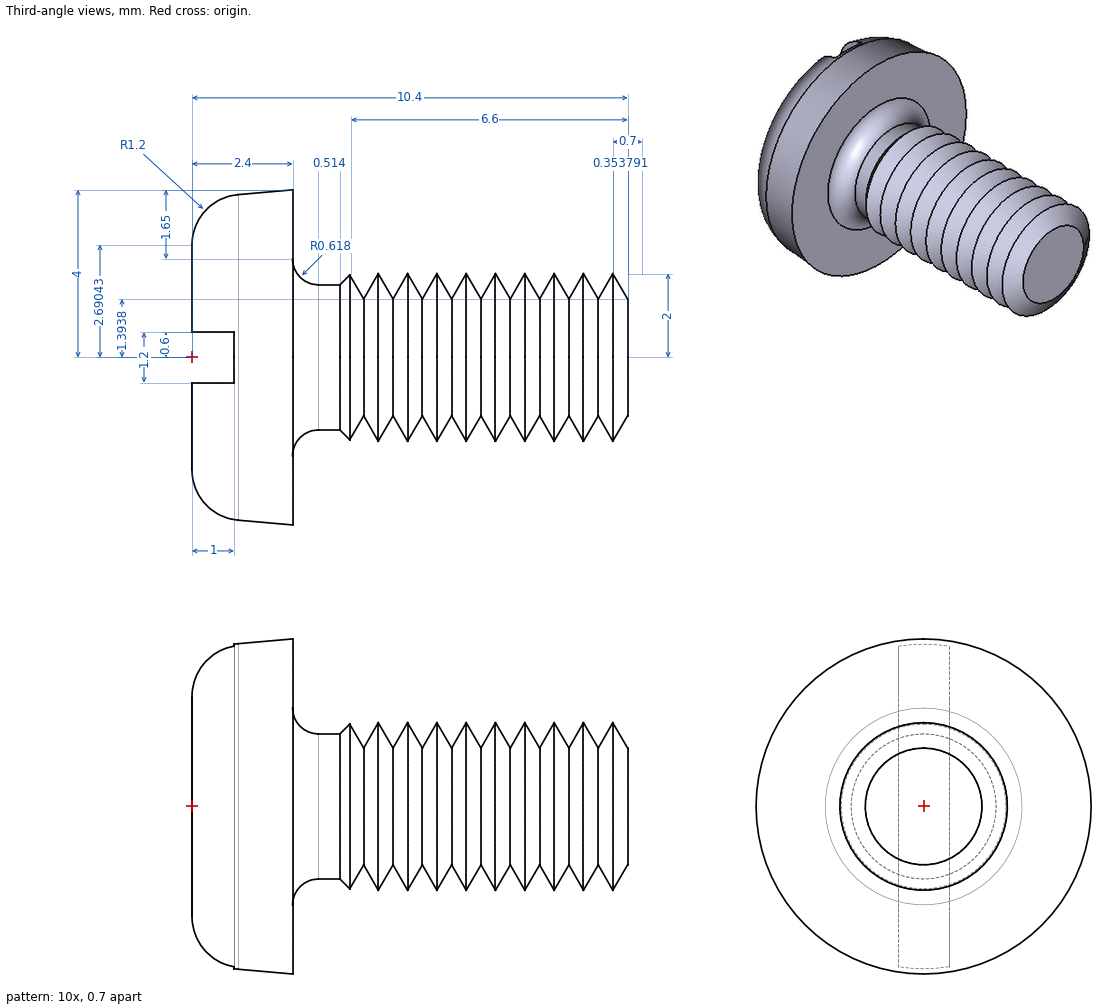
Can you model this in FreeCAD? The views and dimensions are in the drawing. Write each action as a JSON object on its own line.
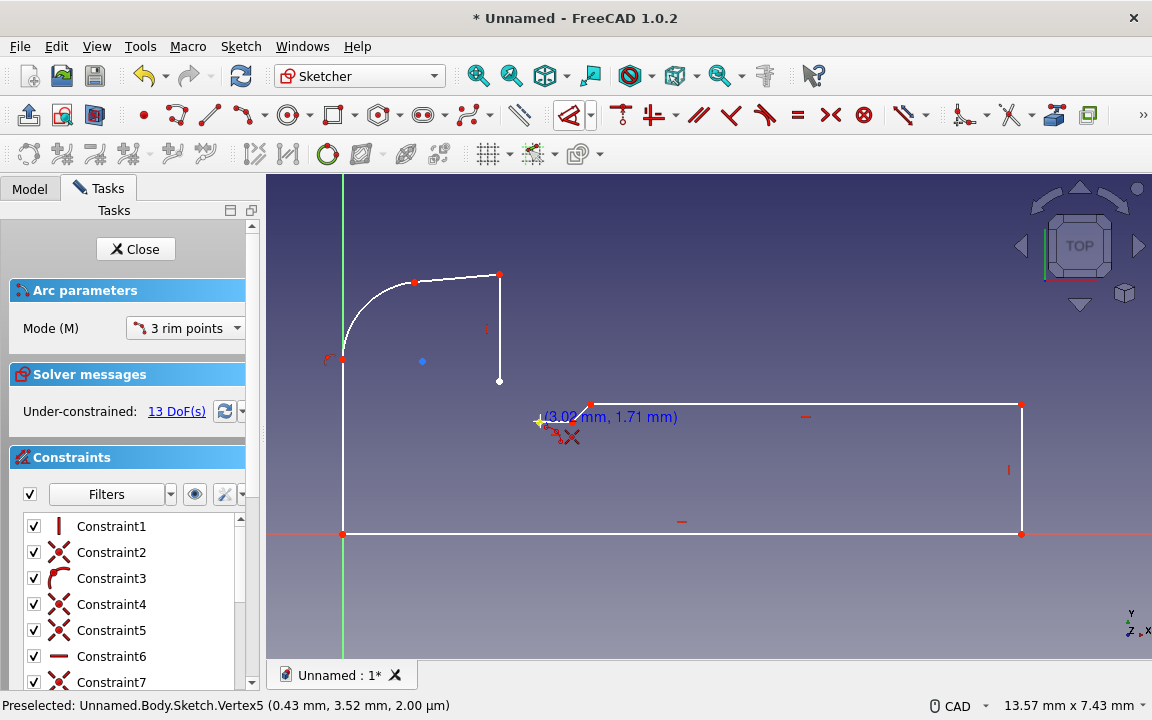
{"action": "left_click", "coordinate": [540, 422]}
{"action": "left_click", "coordinate": [500, 382]}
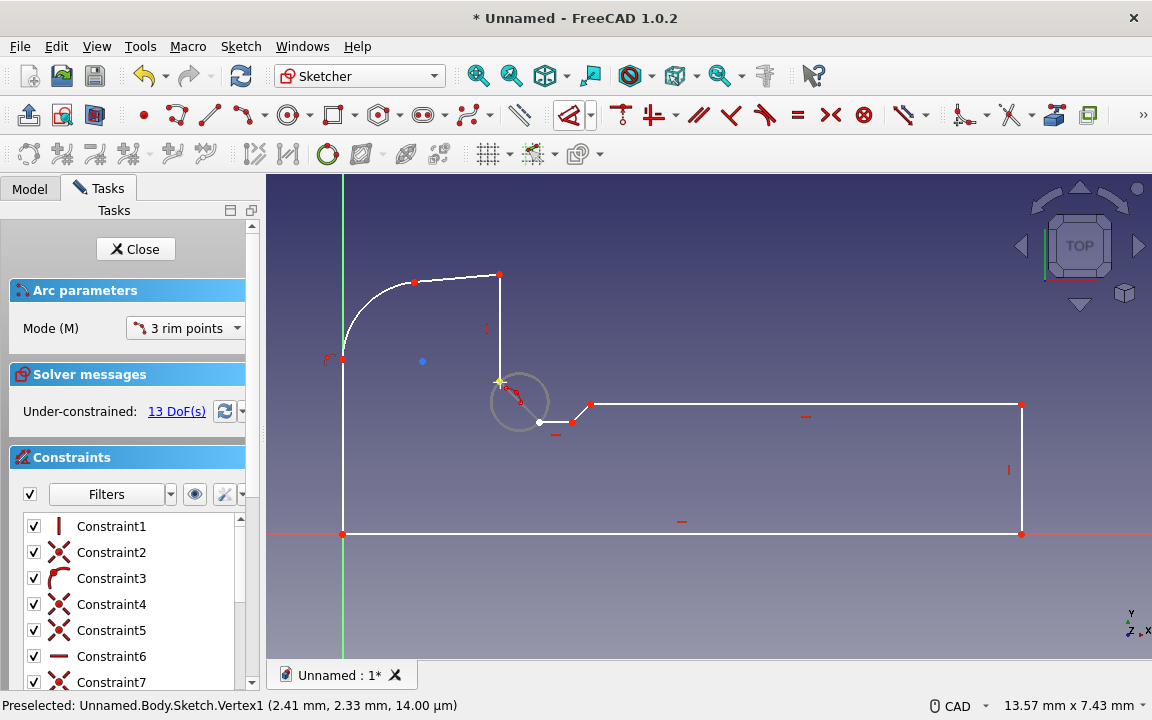
{"action": "scroll", "coordinate": [511, 409], "scroll_direction": "up", "scroll_amount": 2}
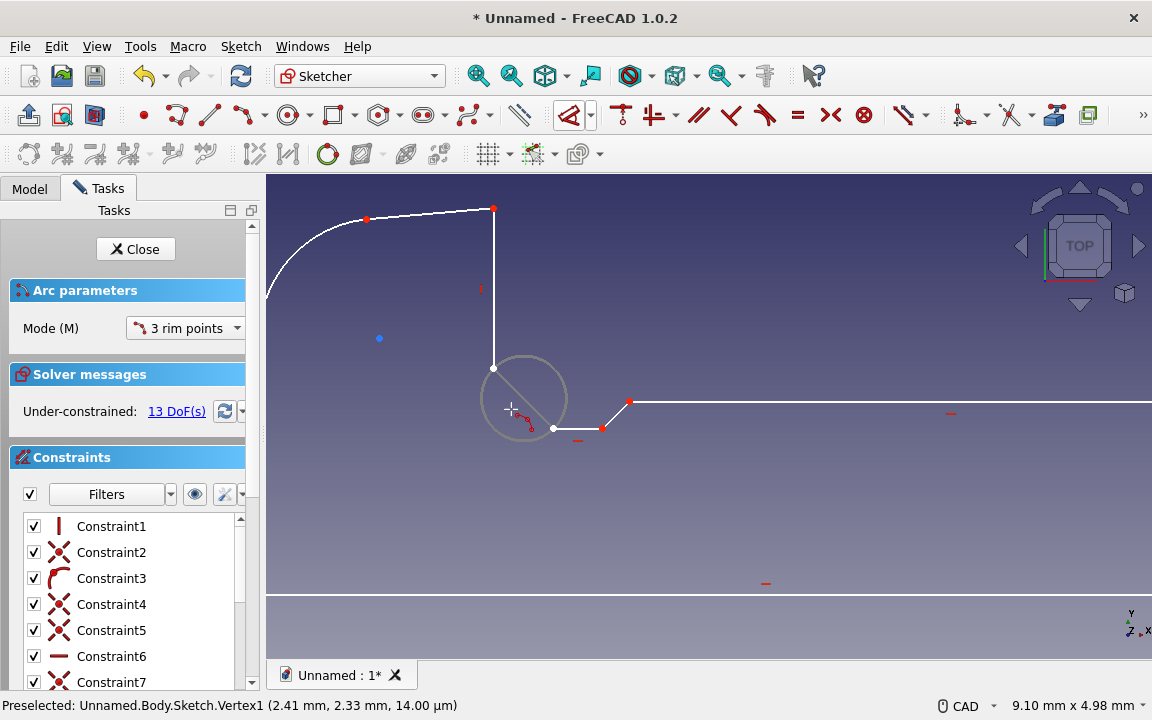
{"action": "left_click", "coordinate": [511, 409]}
{"action": "key", "text": "Escape"}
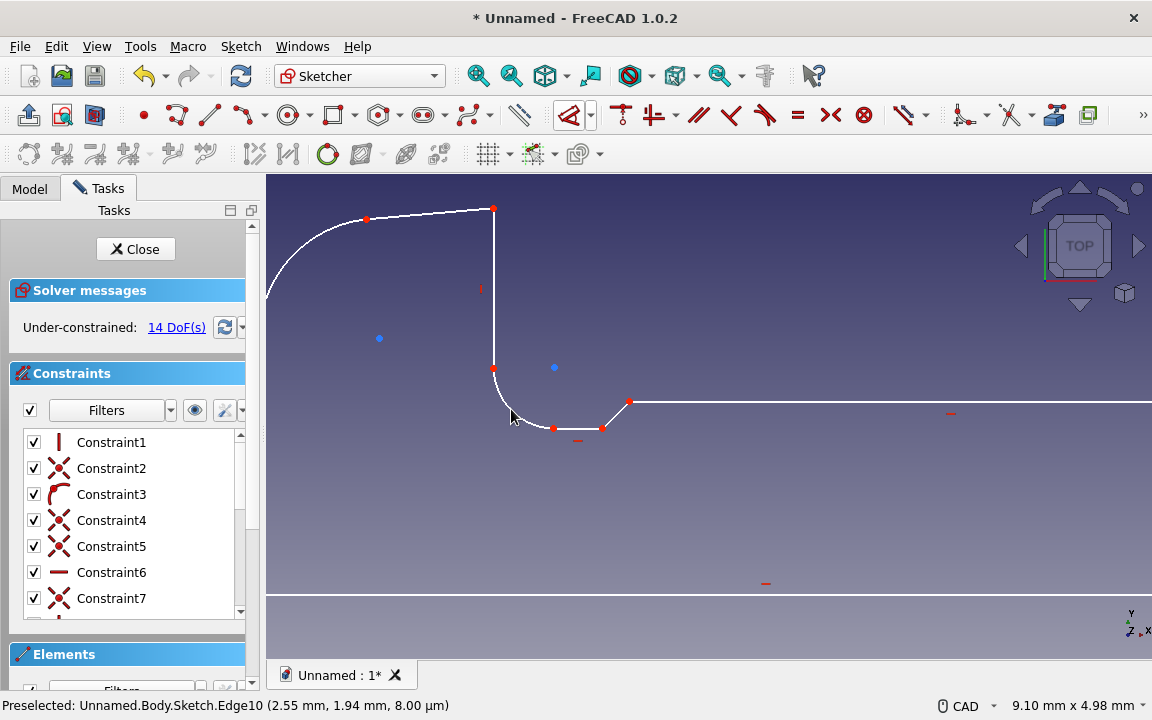
{"action": "left_click", "coordinate": [494, 320]}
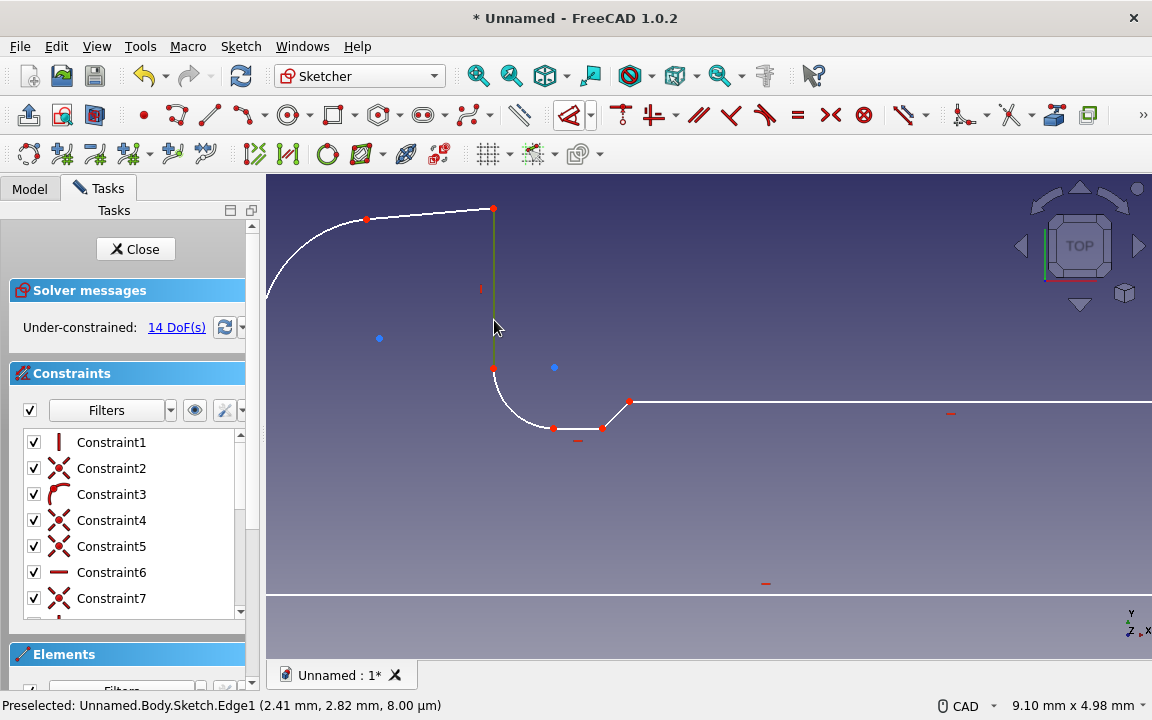
{"action": "left_click", "coordinate": [501, 396]}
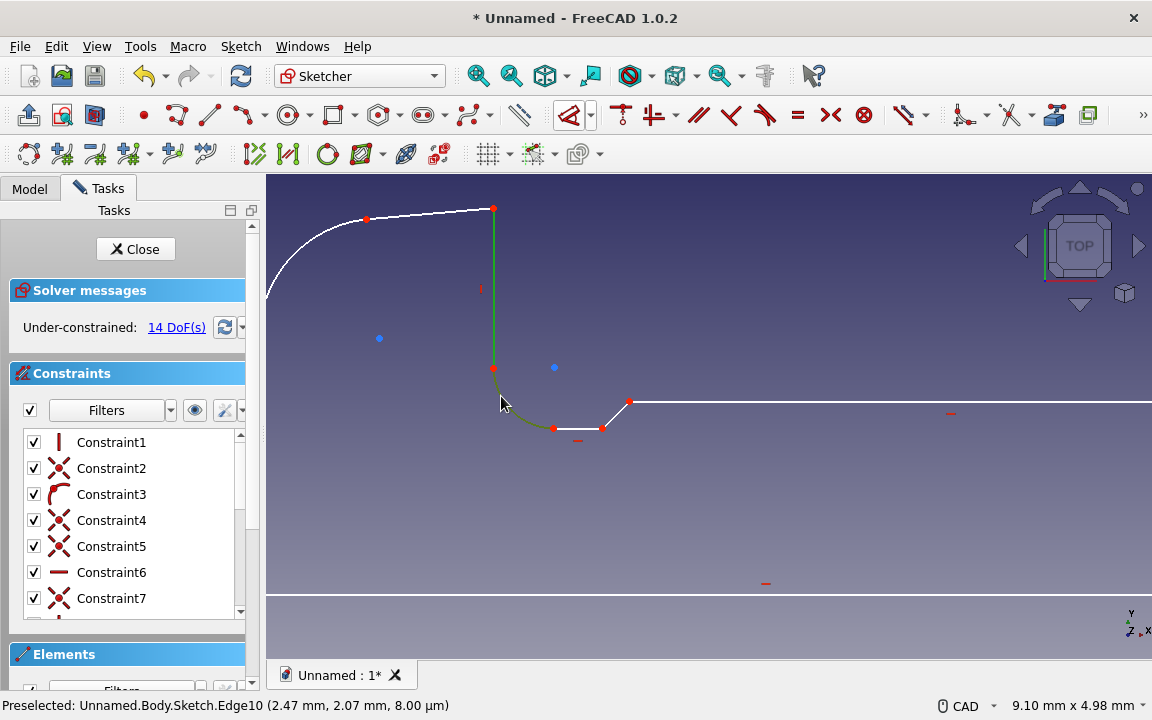
{"action": "left_click", "coordinate": [765, 116]}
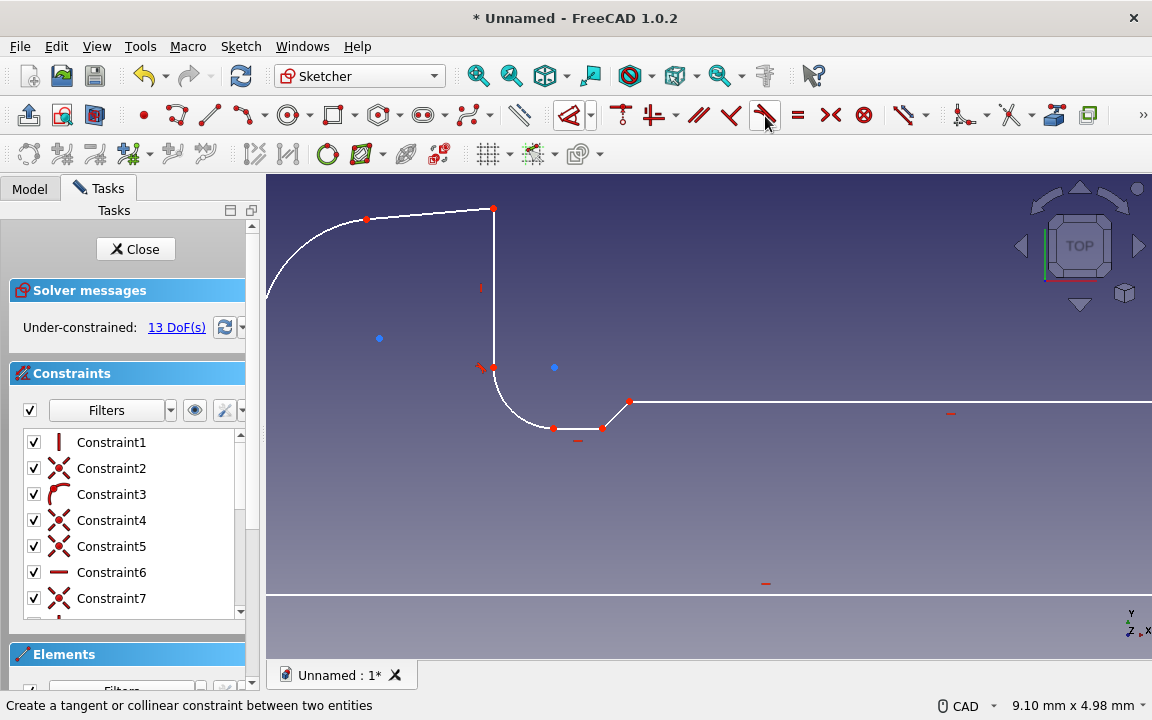
{"action": "left_click", "coordinate": [456, 212]}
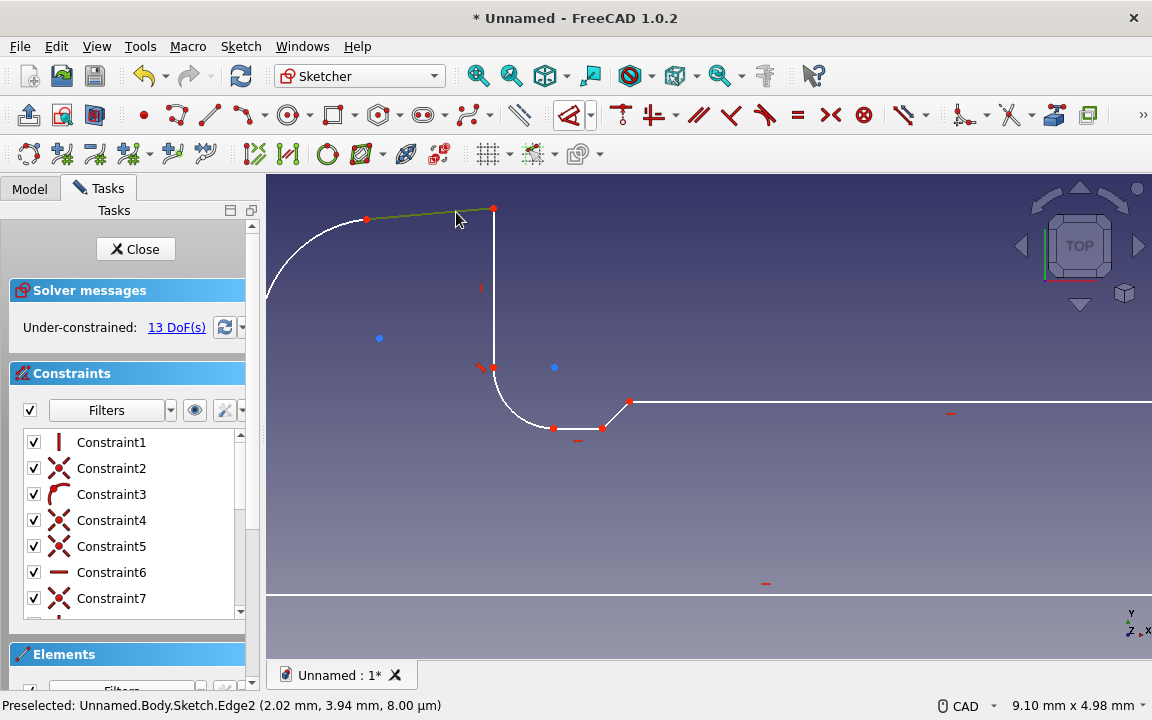
{"action": "left_click", "coordinate": [318, 235]}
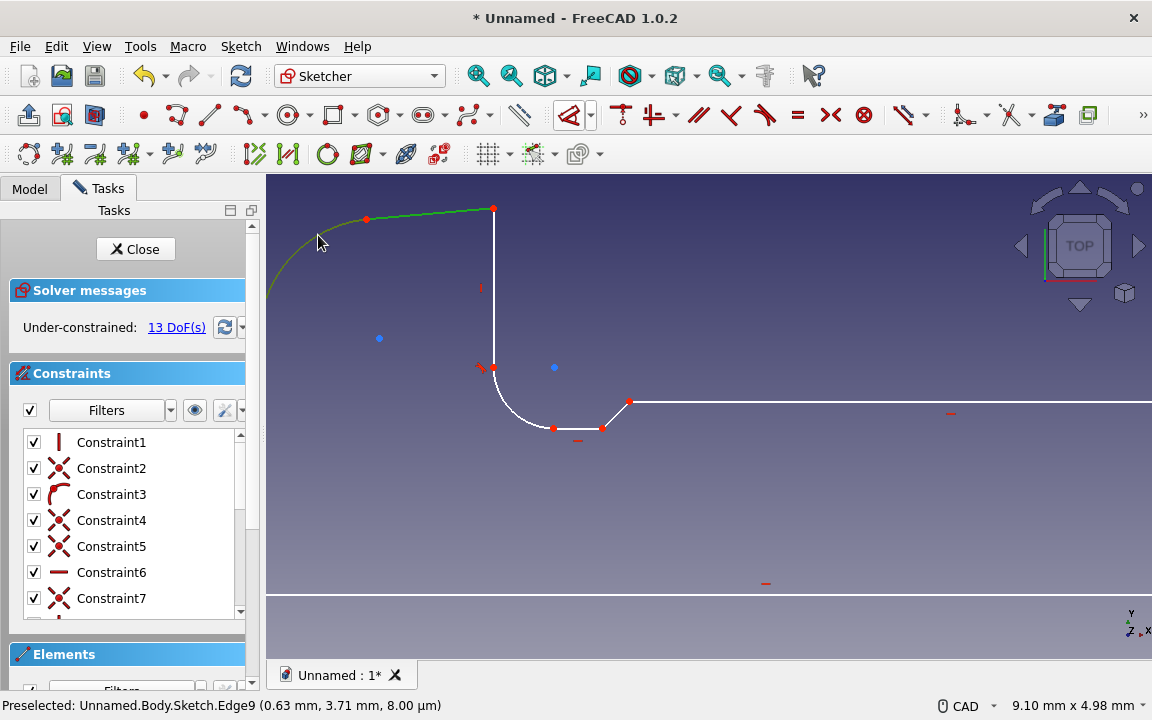
{"action": "left_click", "coordinate": [765, 116]}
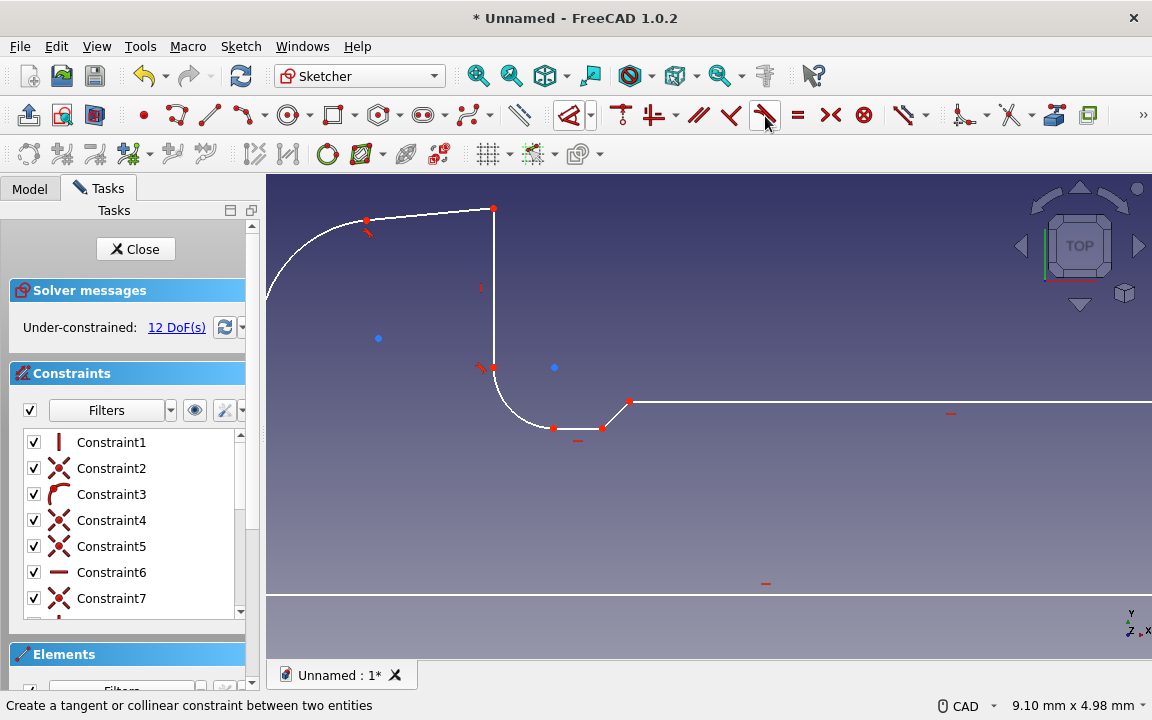
{"action": "scroll", "coordinate": [538, 430], "scroll_direction": "down", "scroll_amount": 4}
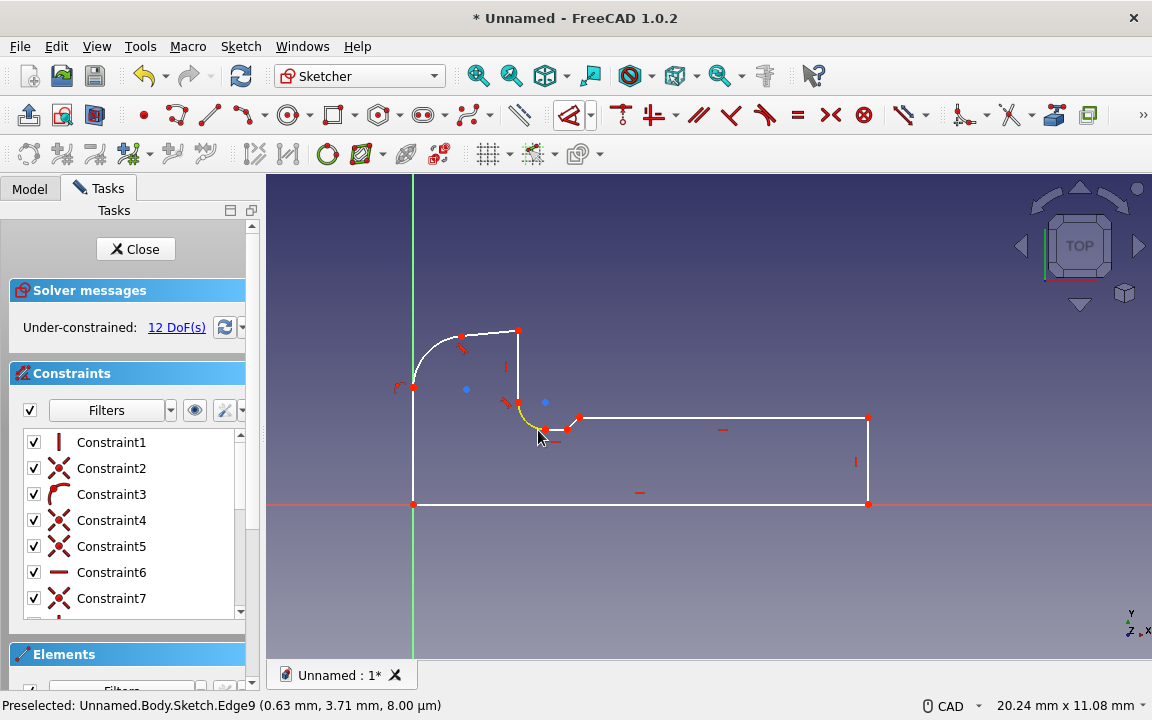
{"action": "left_click", "coordinate": [413, 423]}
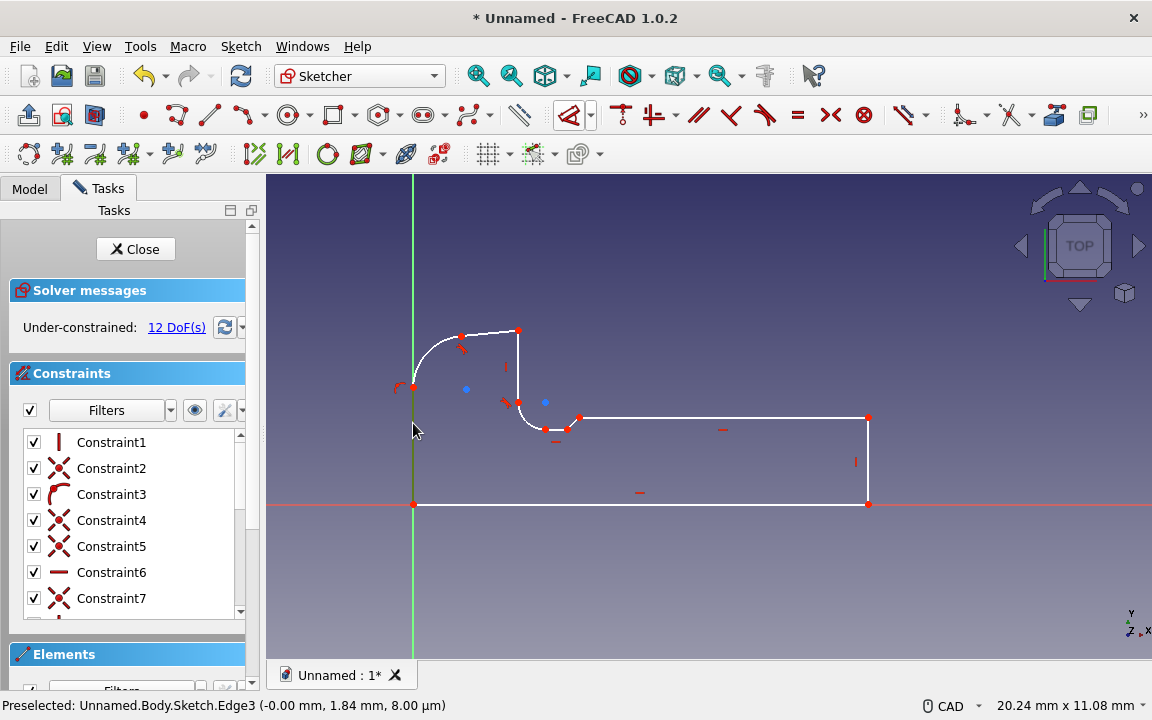
{"action": "left_click", "coordinate": [439, 343]}